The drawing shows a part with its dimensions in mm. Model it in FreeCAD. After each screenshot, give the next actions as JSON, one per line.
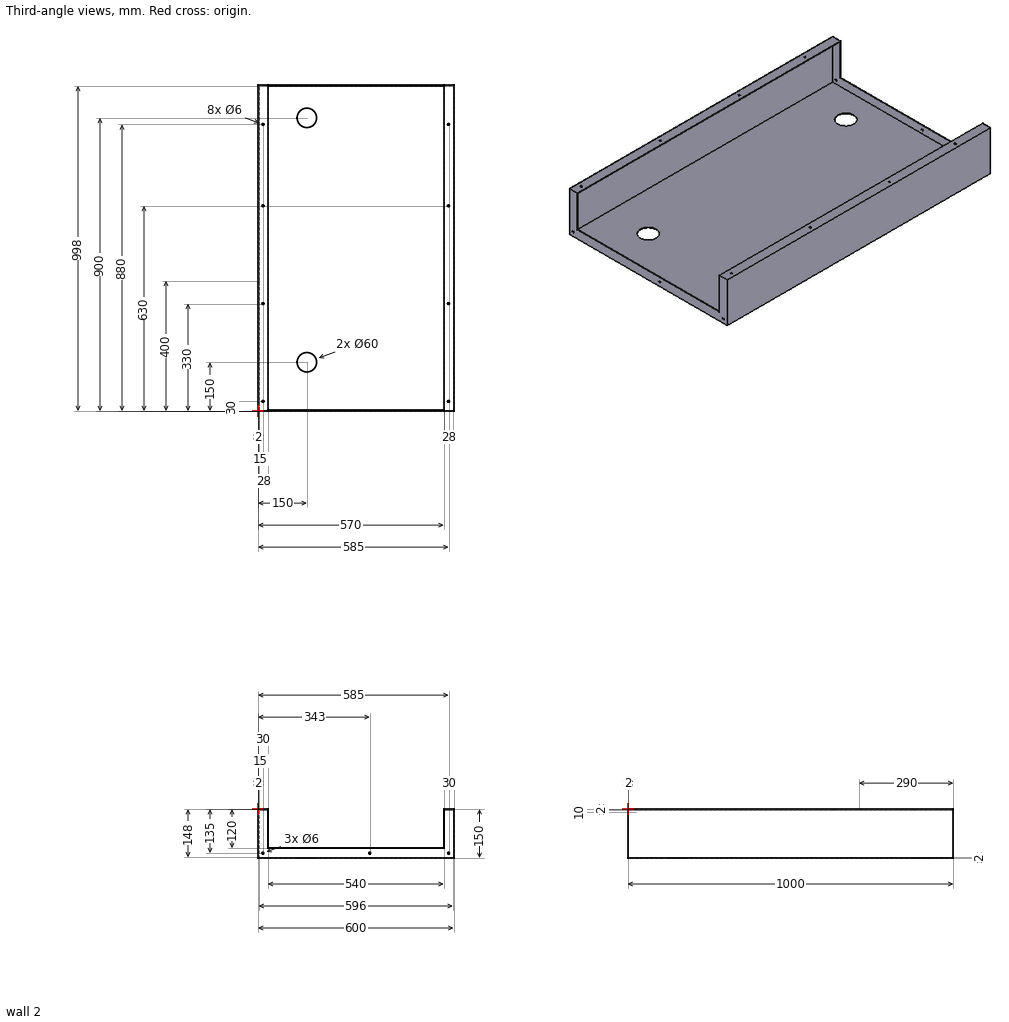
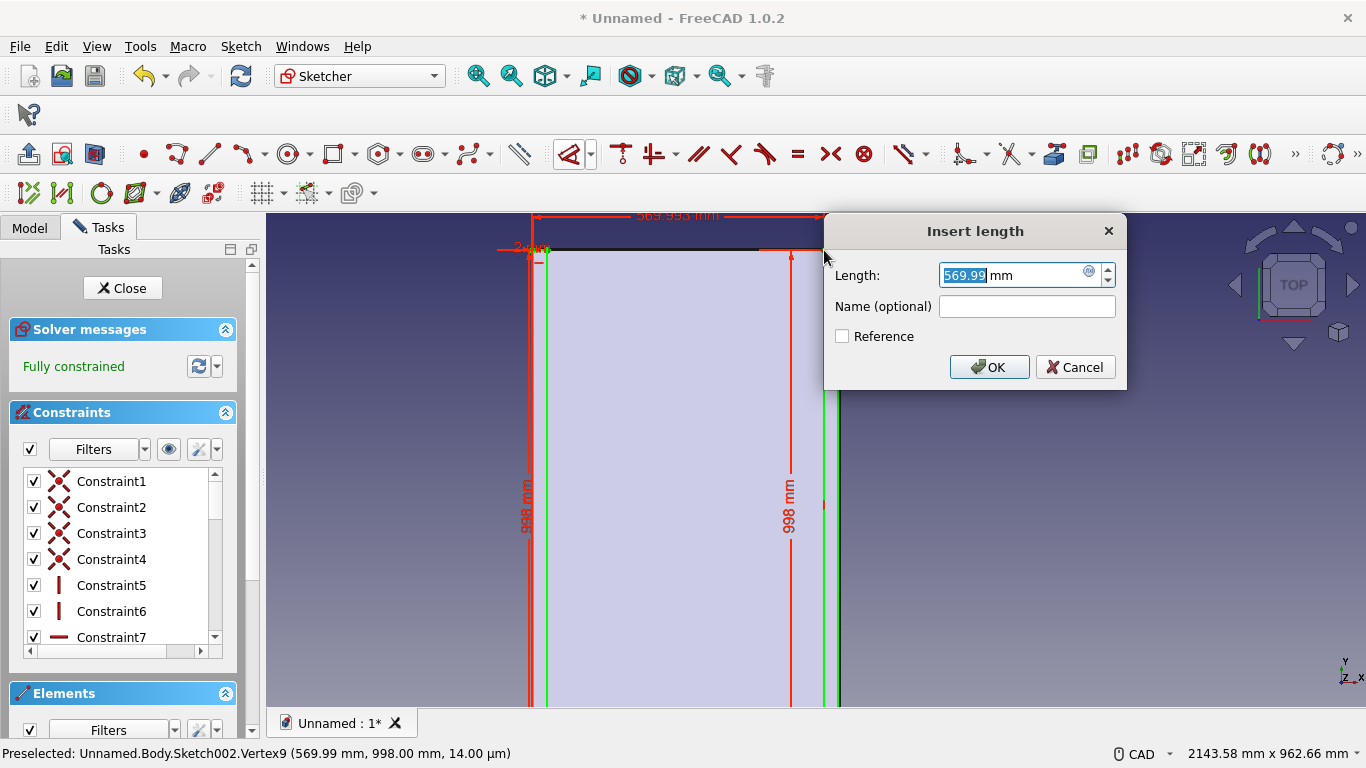
{"action": "type", "text": "570"}
{"action": "key", "text": "Return"}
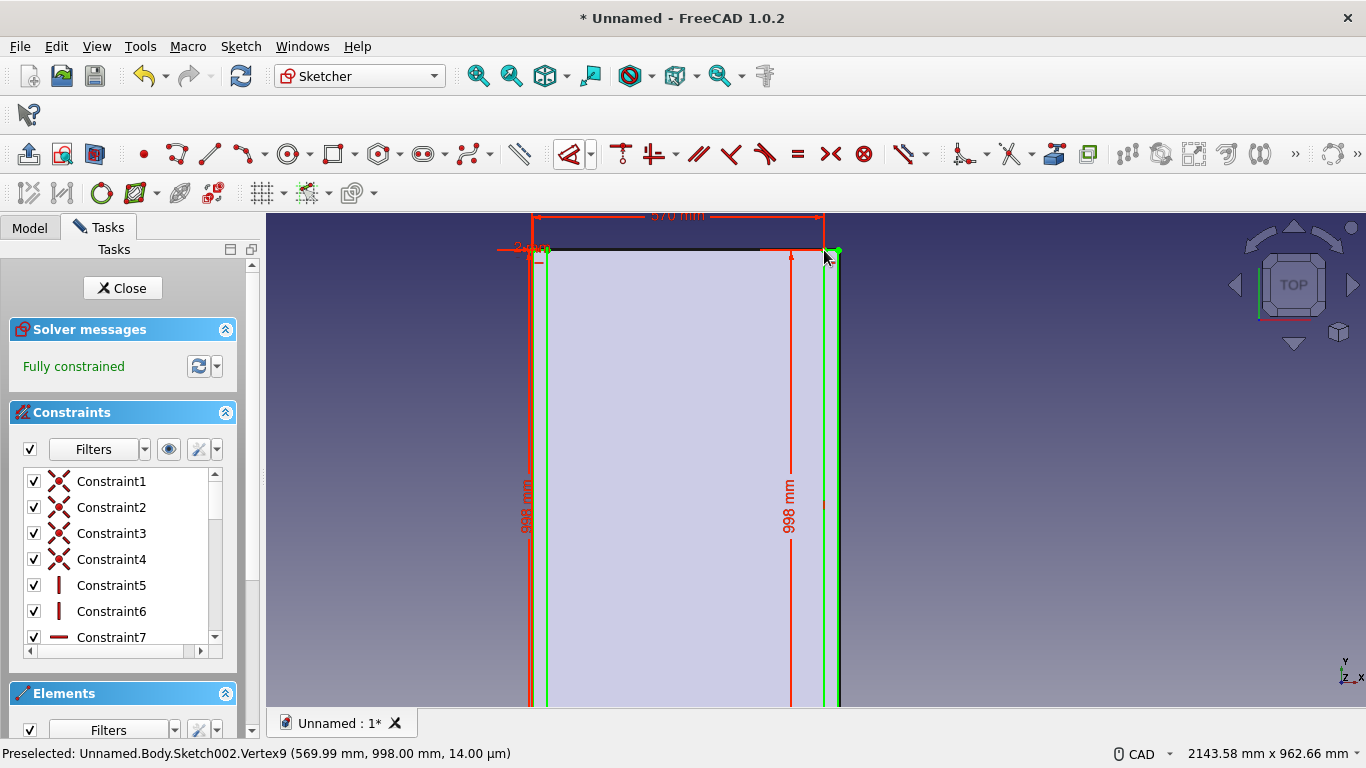
{"action": "left_click", "coordinate": [123, 288]}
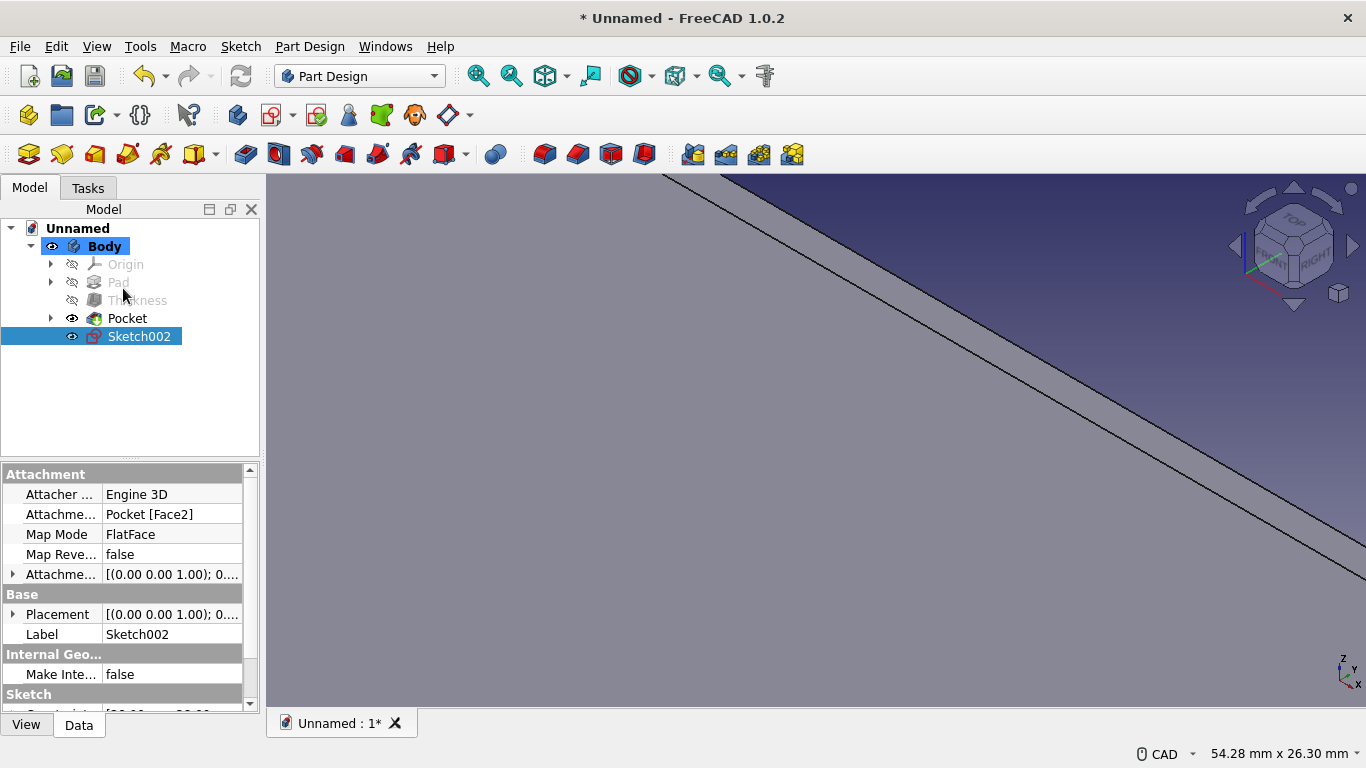
{"action": "left_click", "coordinate": [29, 154]}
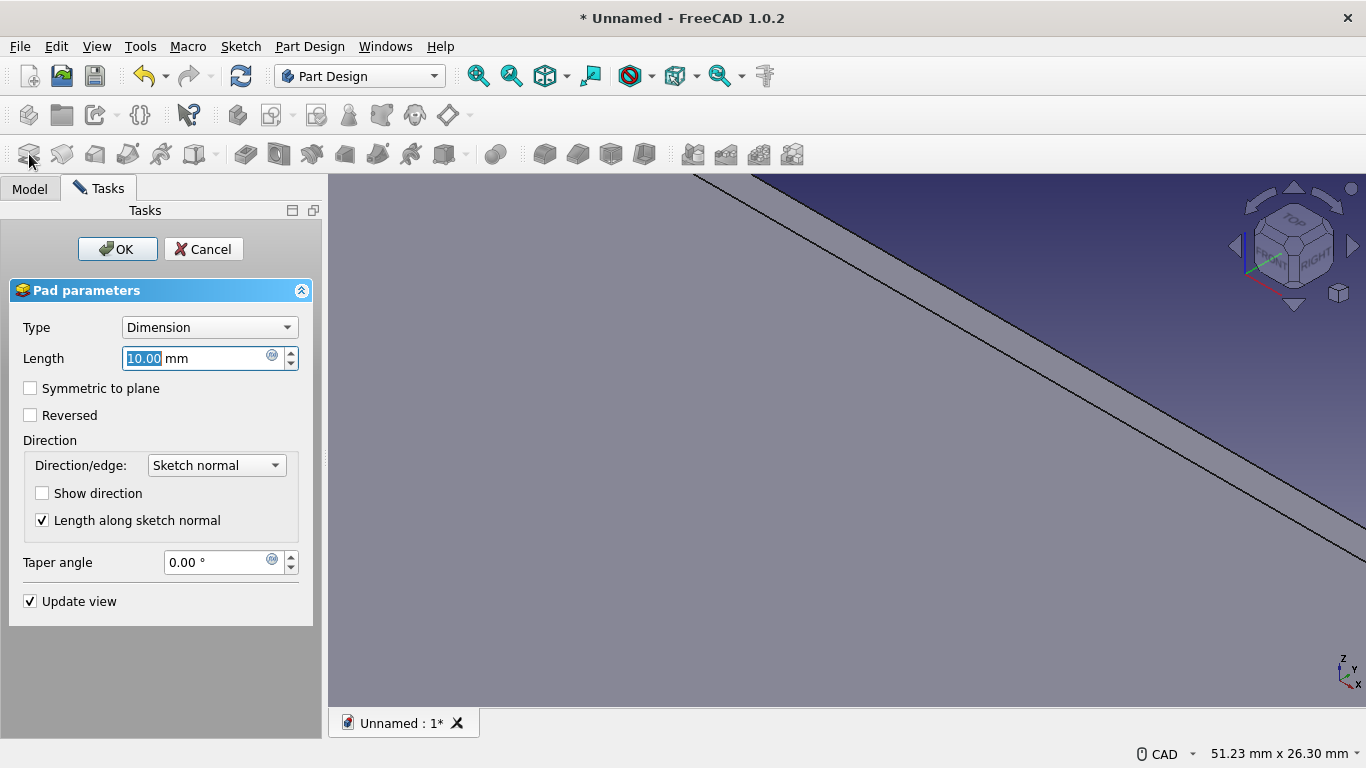
{"action": "type", "text": "2"}
{"action": "key", "text": "Tab"}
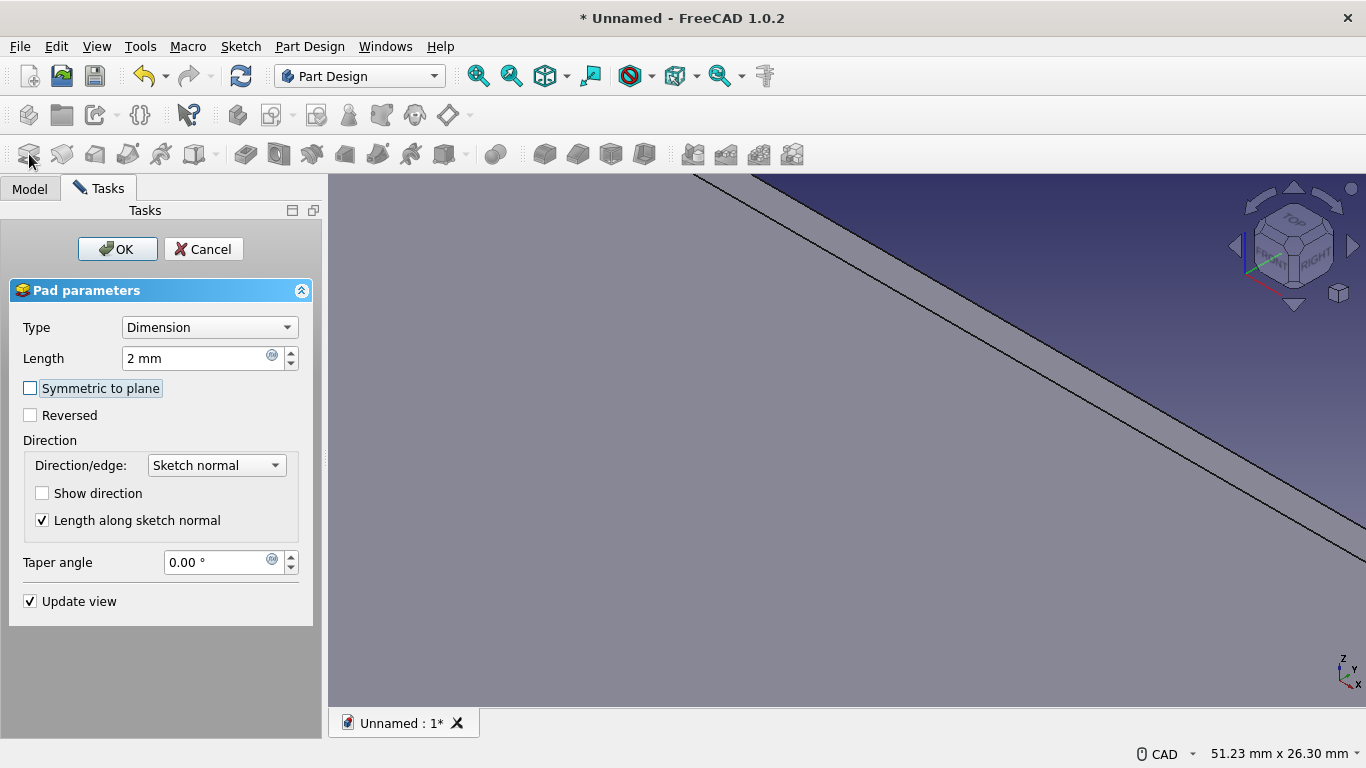
{"action": "left_click", "coordinate": [31, 415]}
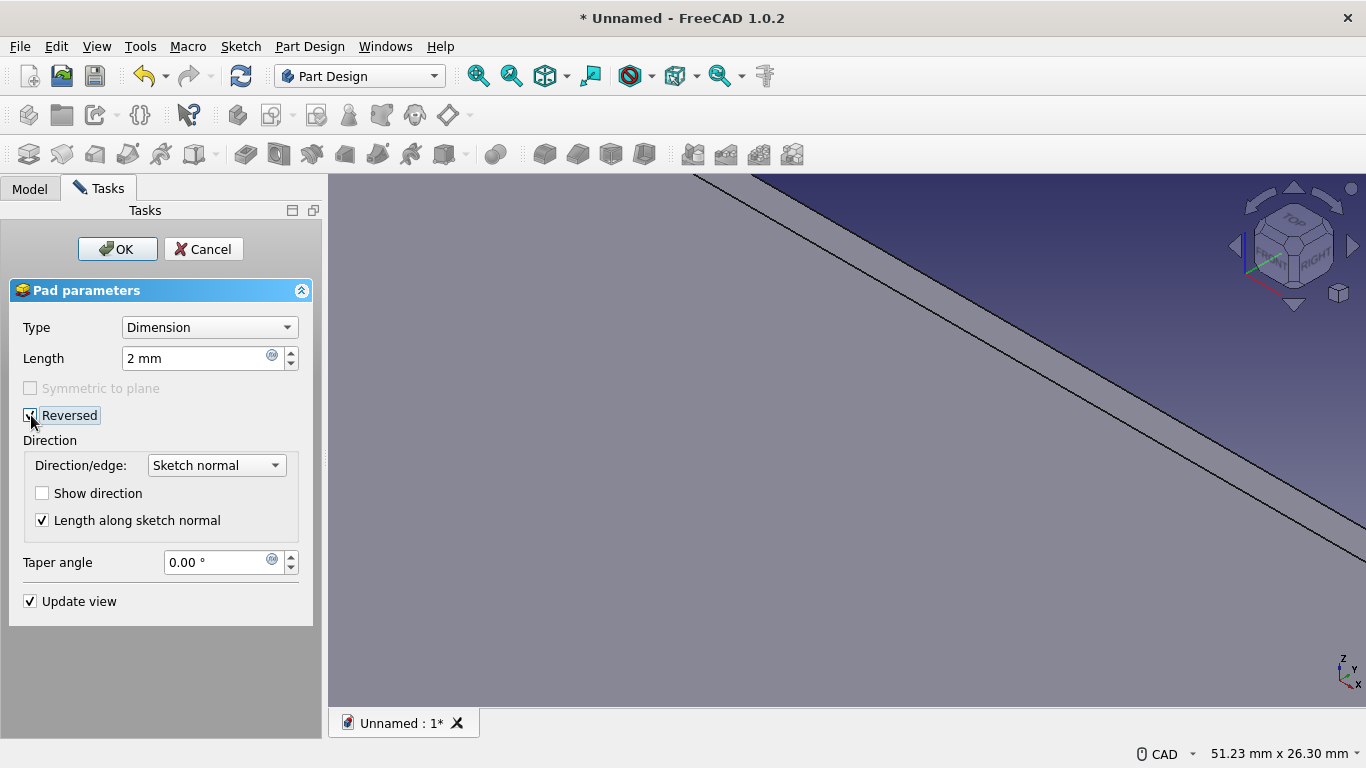
{"action": "left_click", "coordinate": [118, 249]}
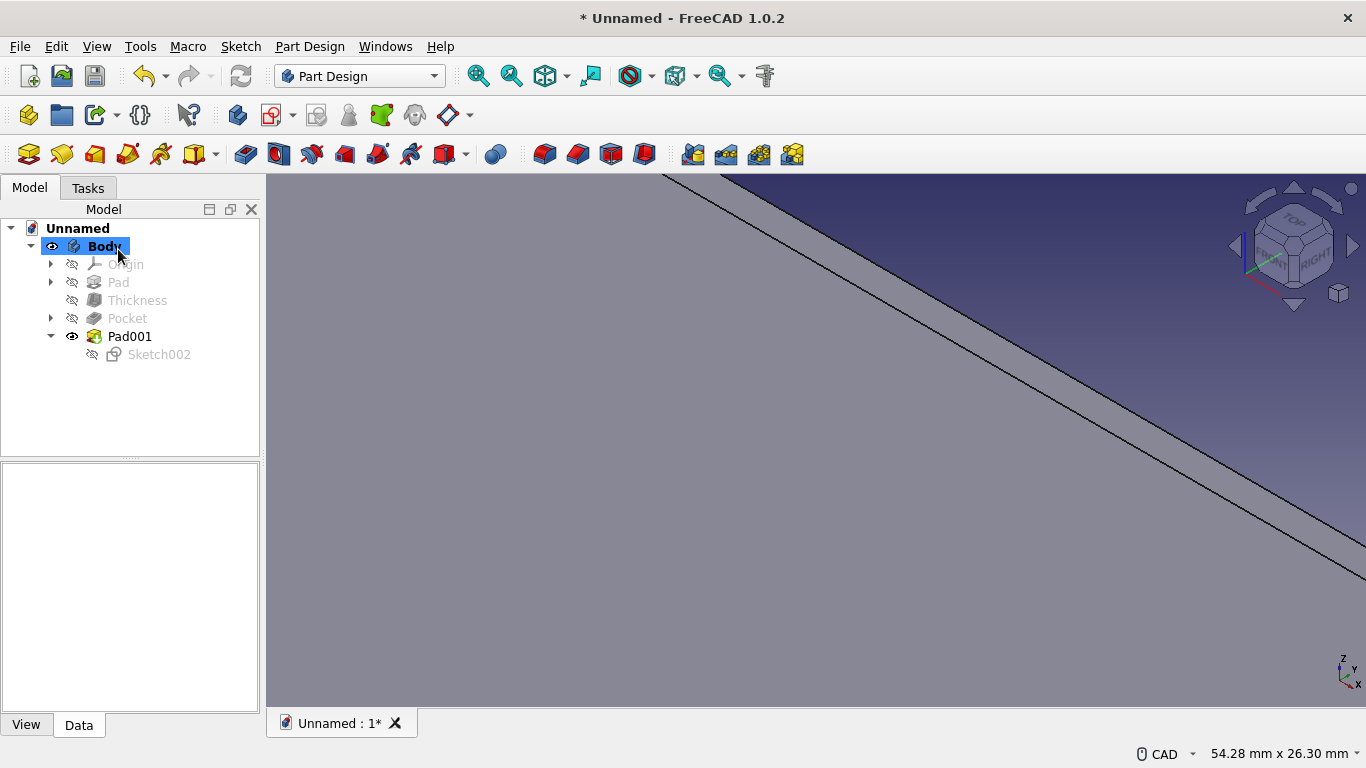
{"action": "left_click", "coordinate": [479, 76]}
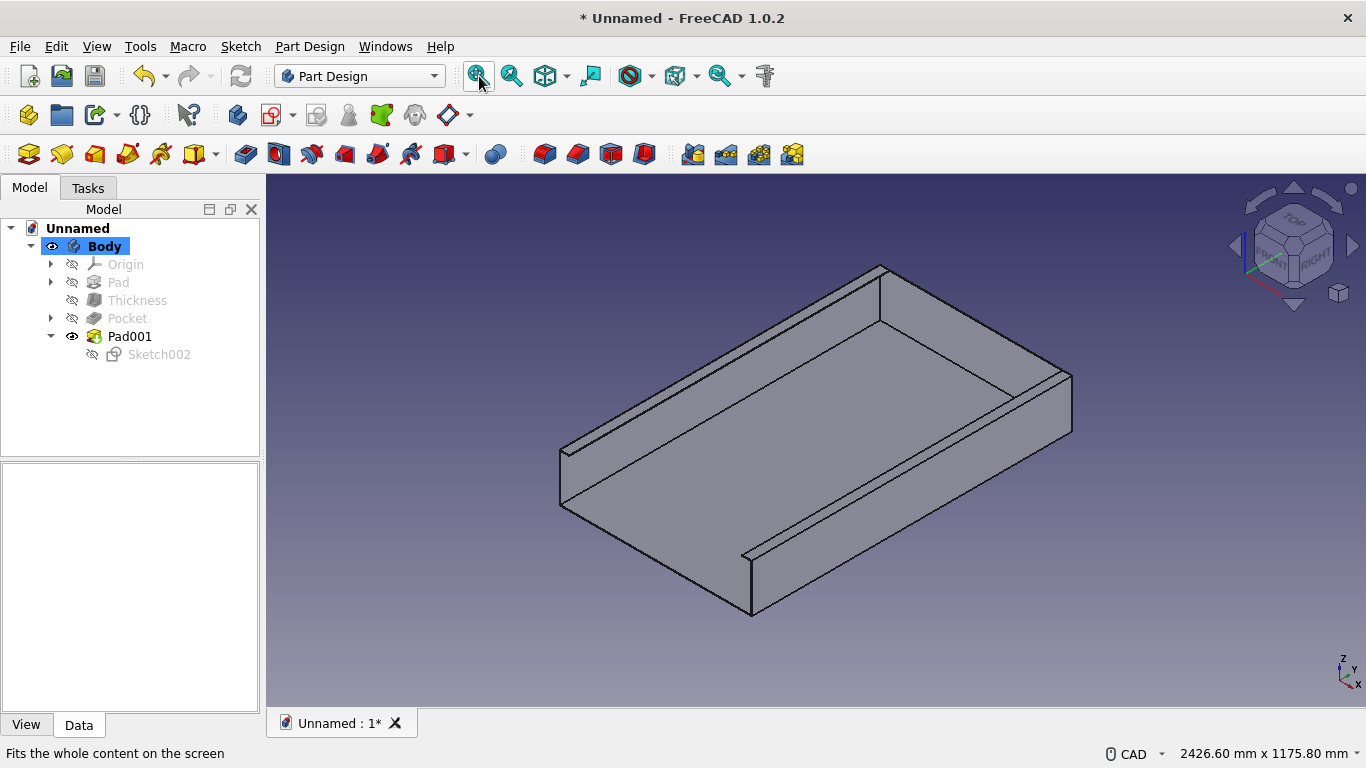
{"action": "key", "text": "5"}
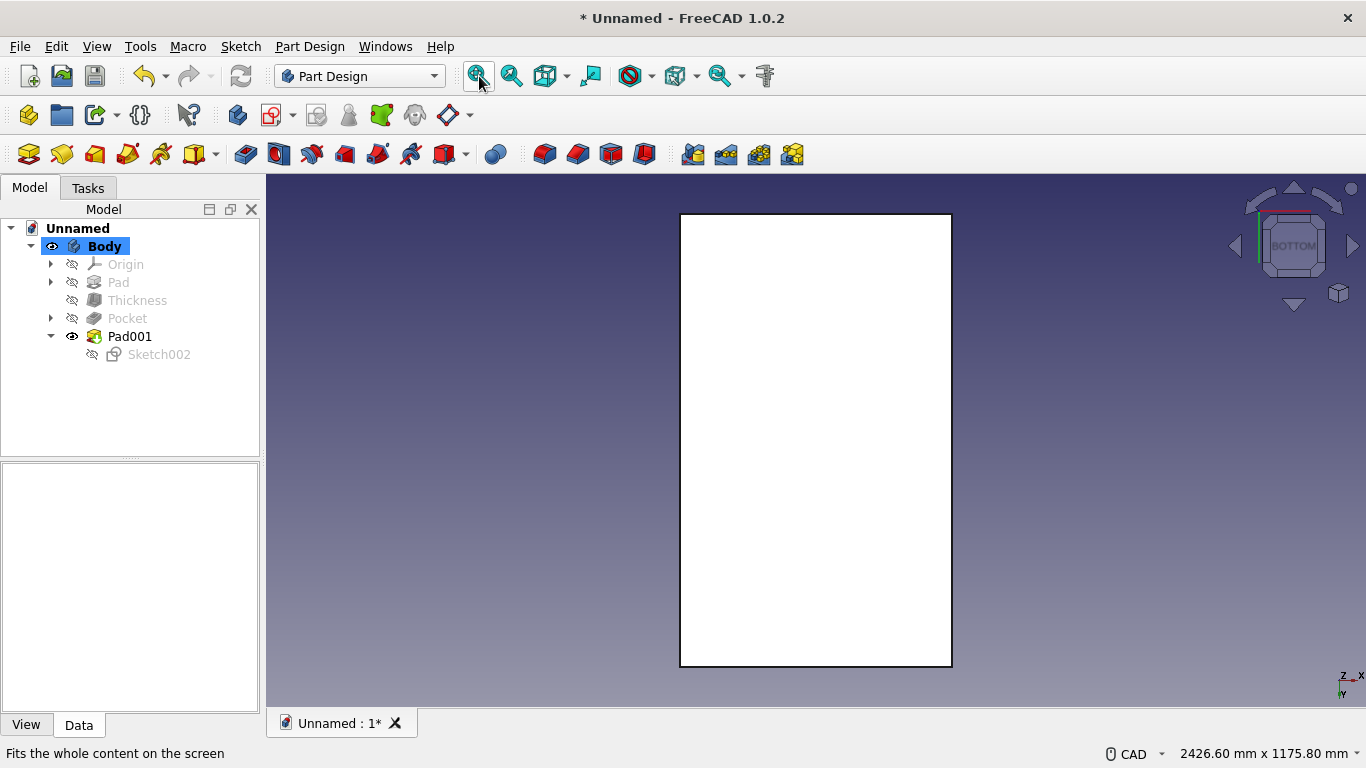
{"action": "left_click", "coordinate": [816, 504]}